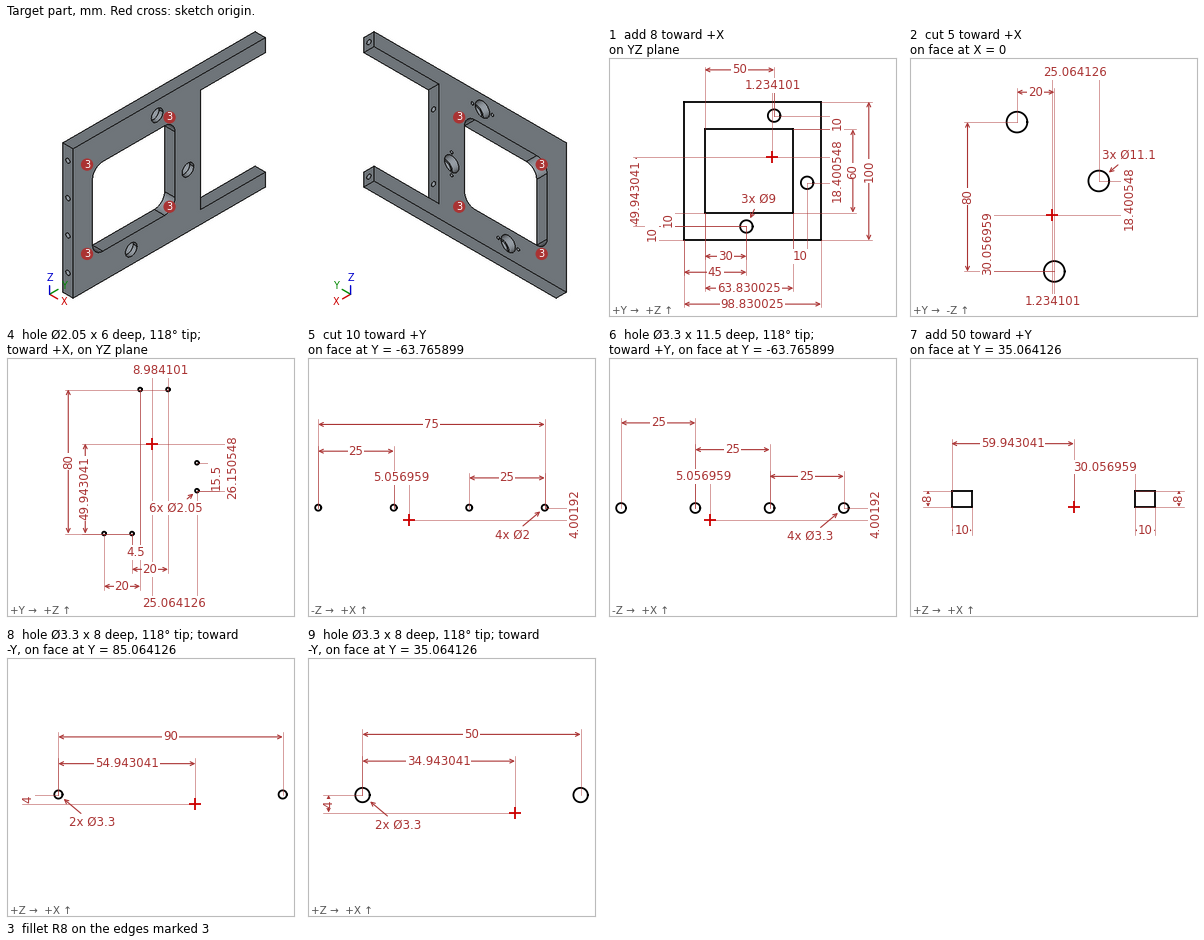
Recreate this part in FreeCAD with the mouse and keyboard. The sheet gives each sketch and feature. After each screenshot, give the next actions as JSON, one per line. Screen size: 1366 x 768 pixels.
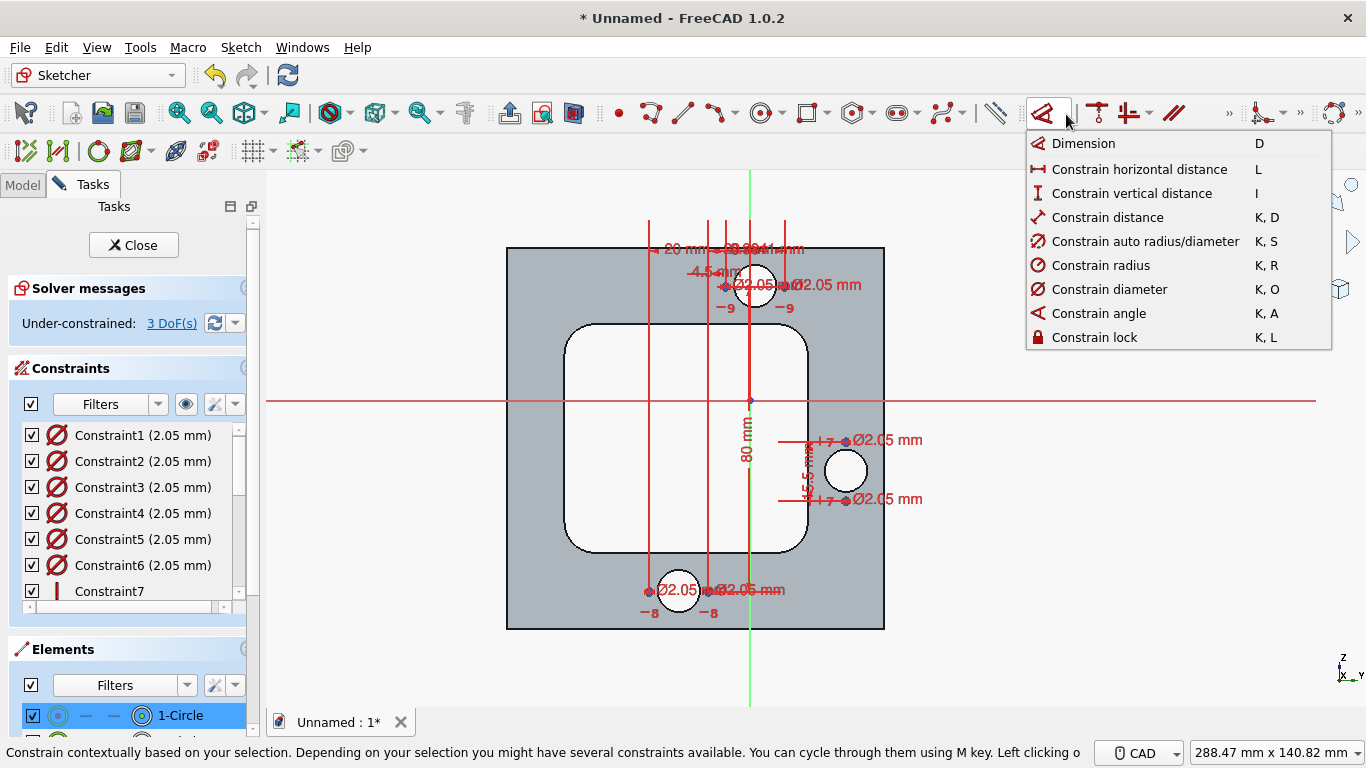
{"action": "left_click", "coordinate": [1179, 169]}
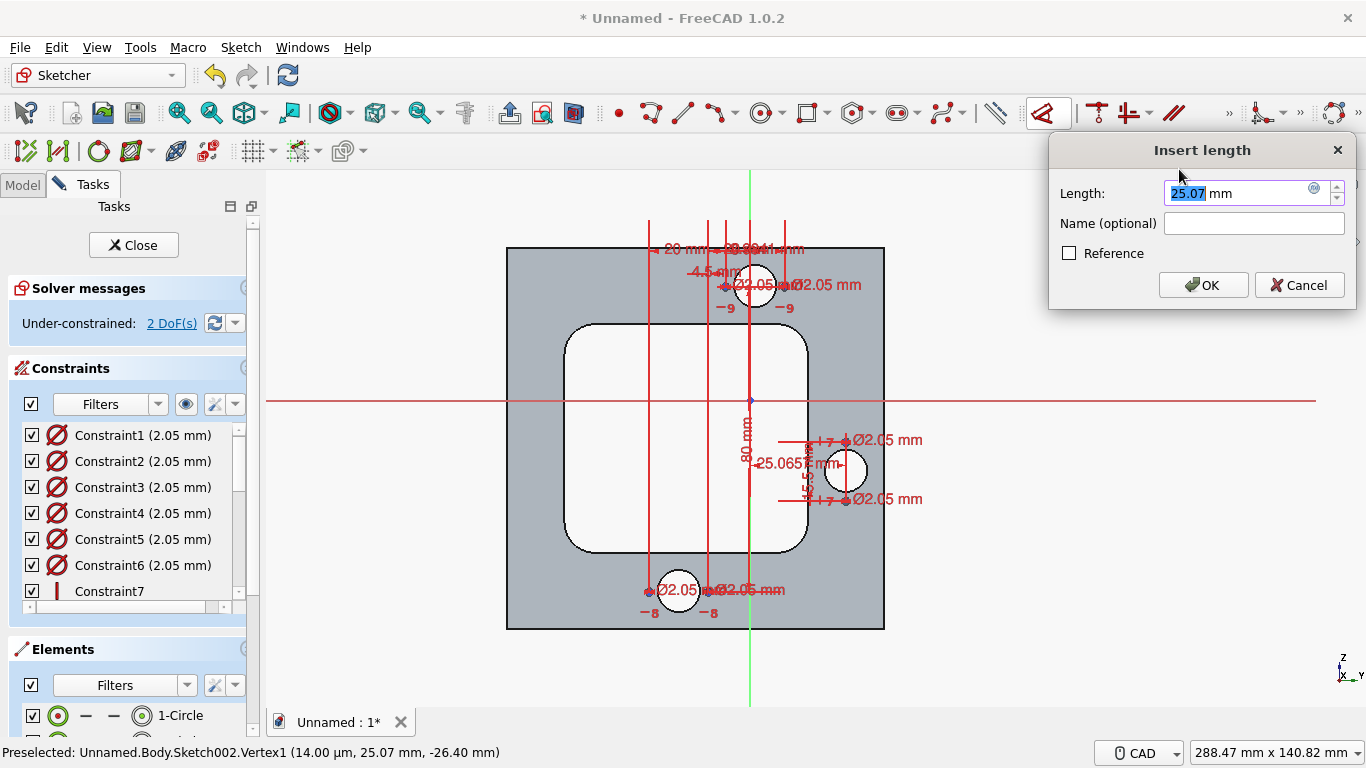
{"action": "type", "text": "25.064126"}
{"action": "key", "text": "Return"}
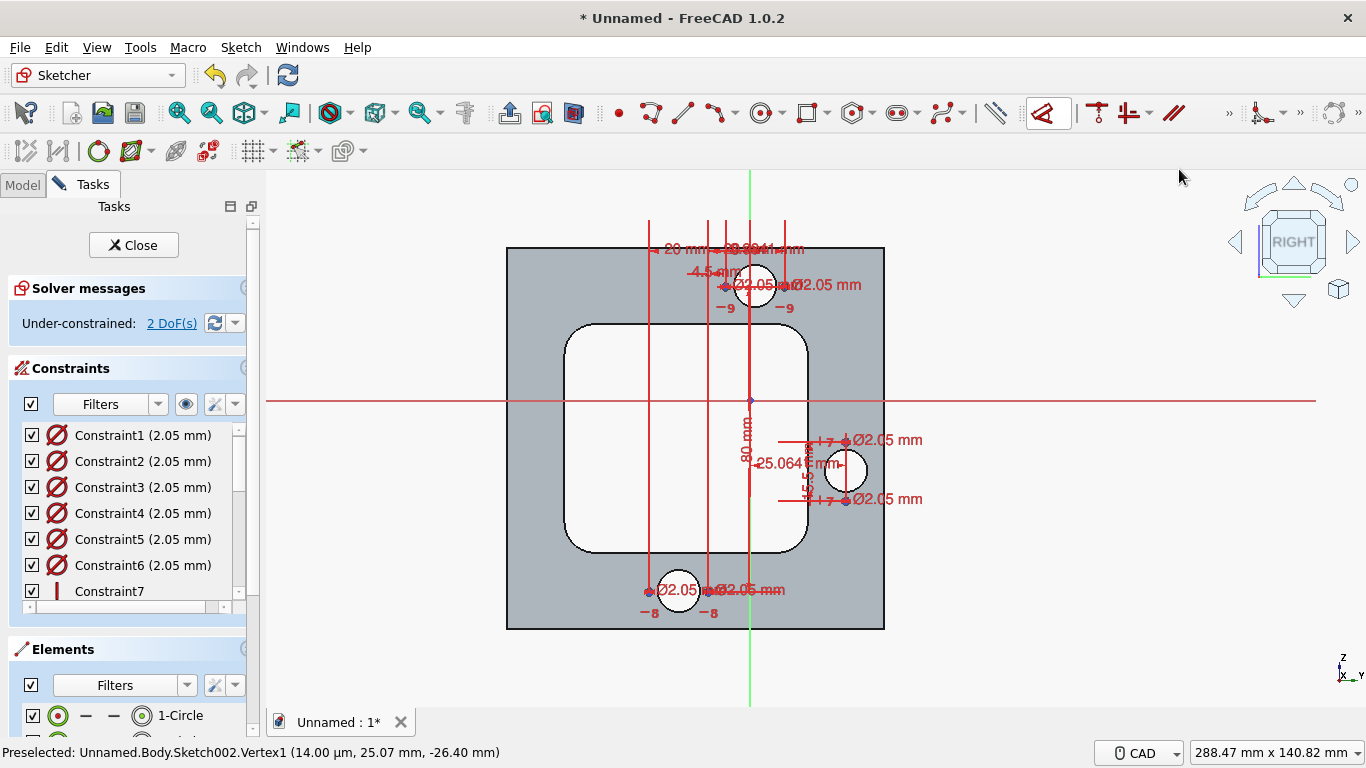
{"action": "left_click", "coordinate": [846, 501]}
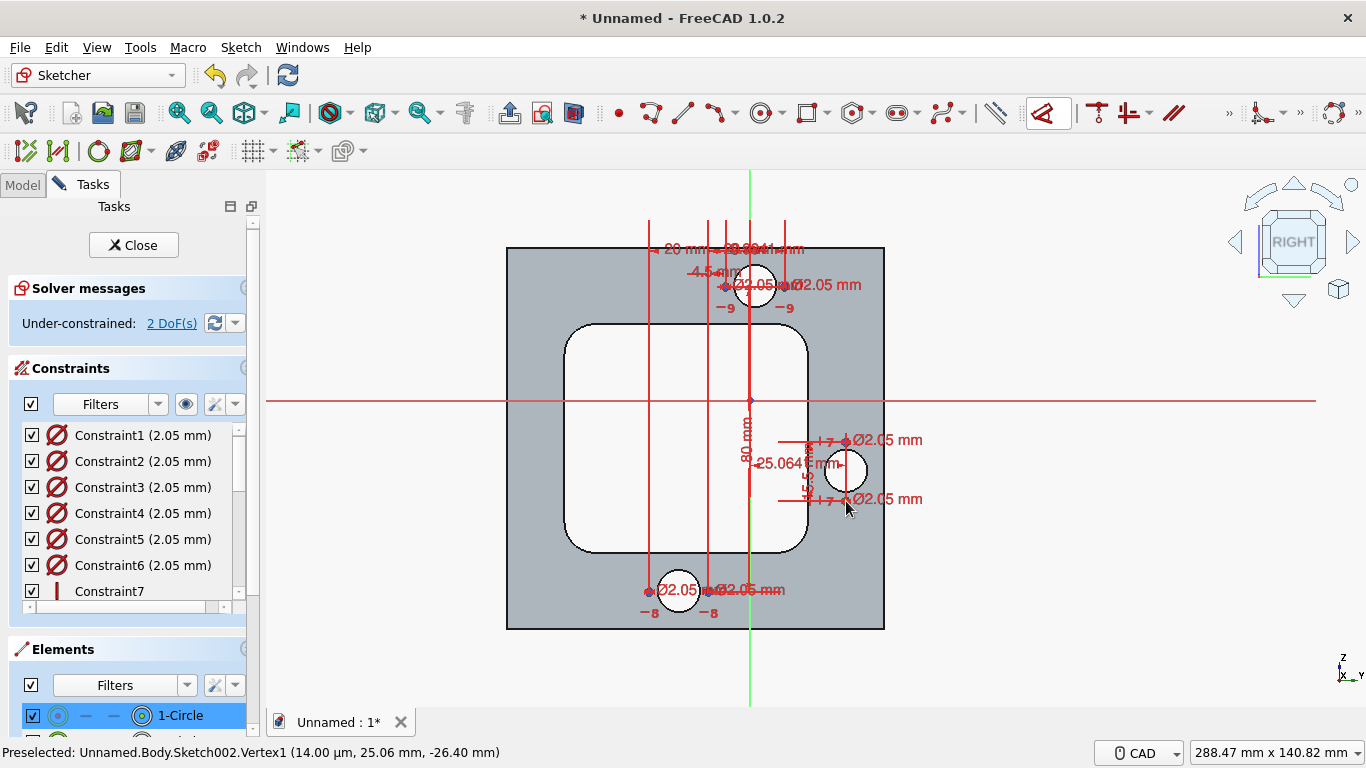
{"action": "key", "text": "i"}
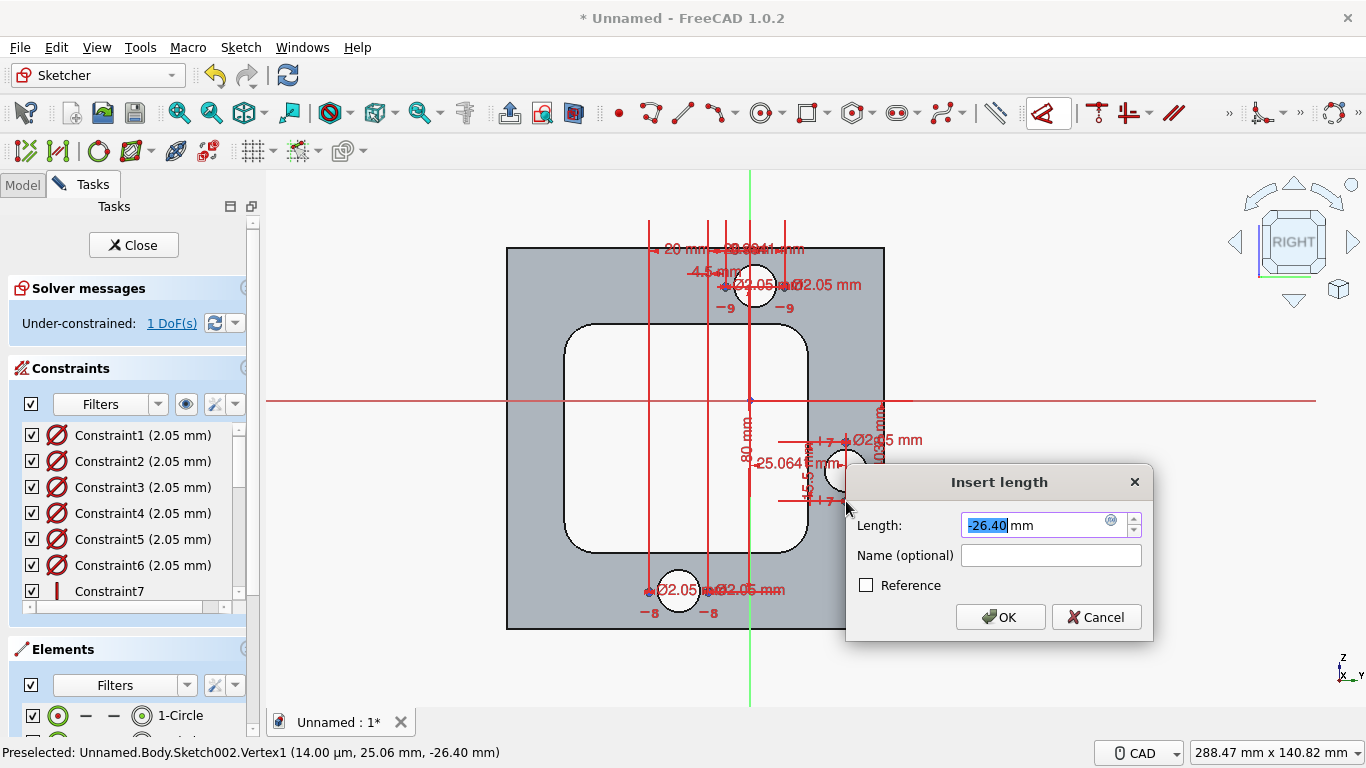
{"action": "type", "text": "-26.150548"}
{"action": "key", "text": "Return"}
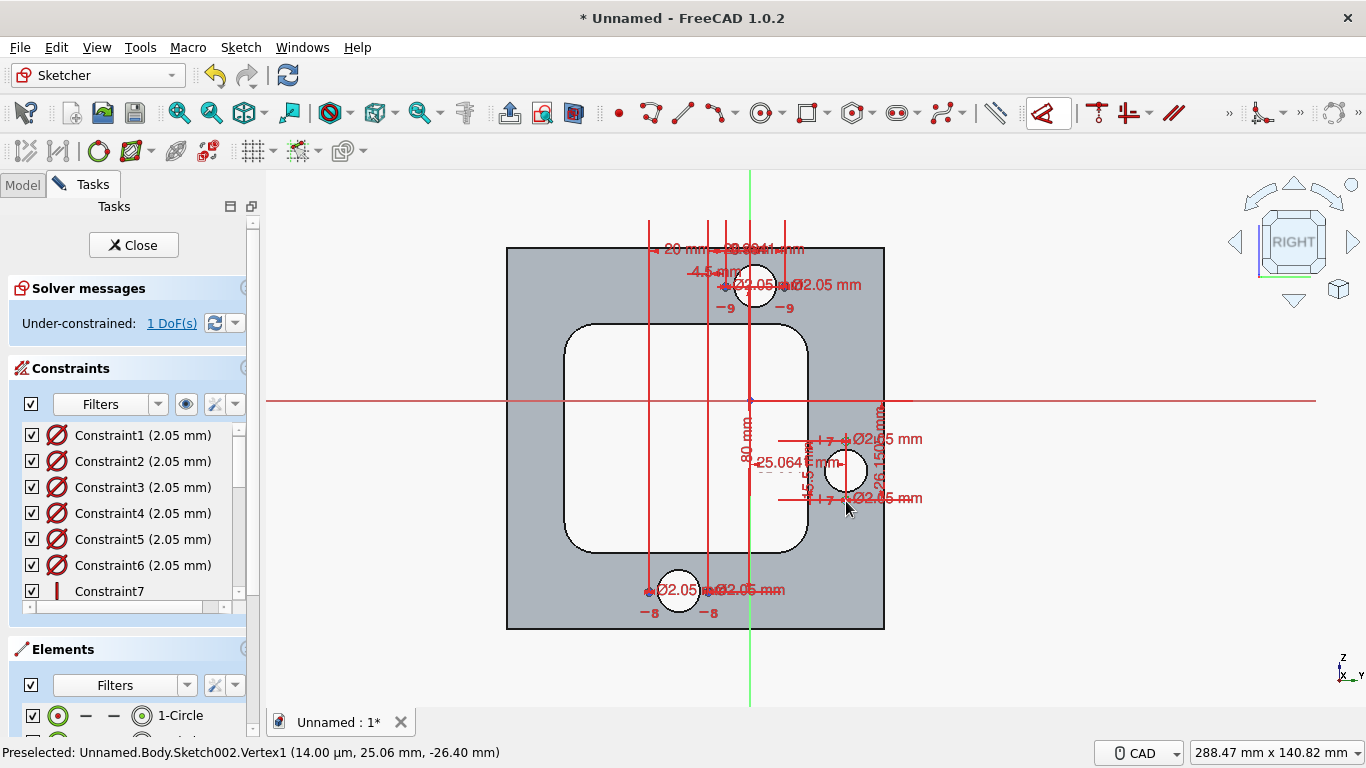
{"action": "left_click", "coordinate": [708, 592]}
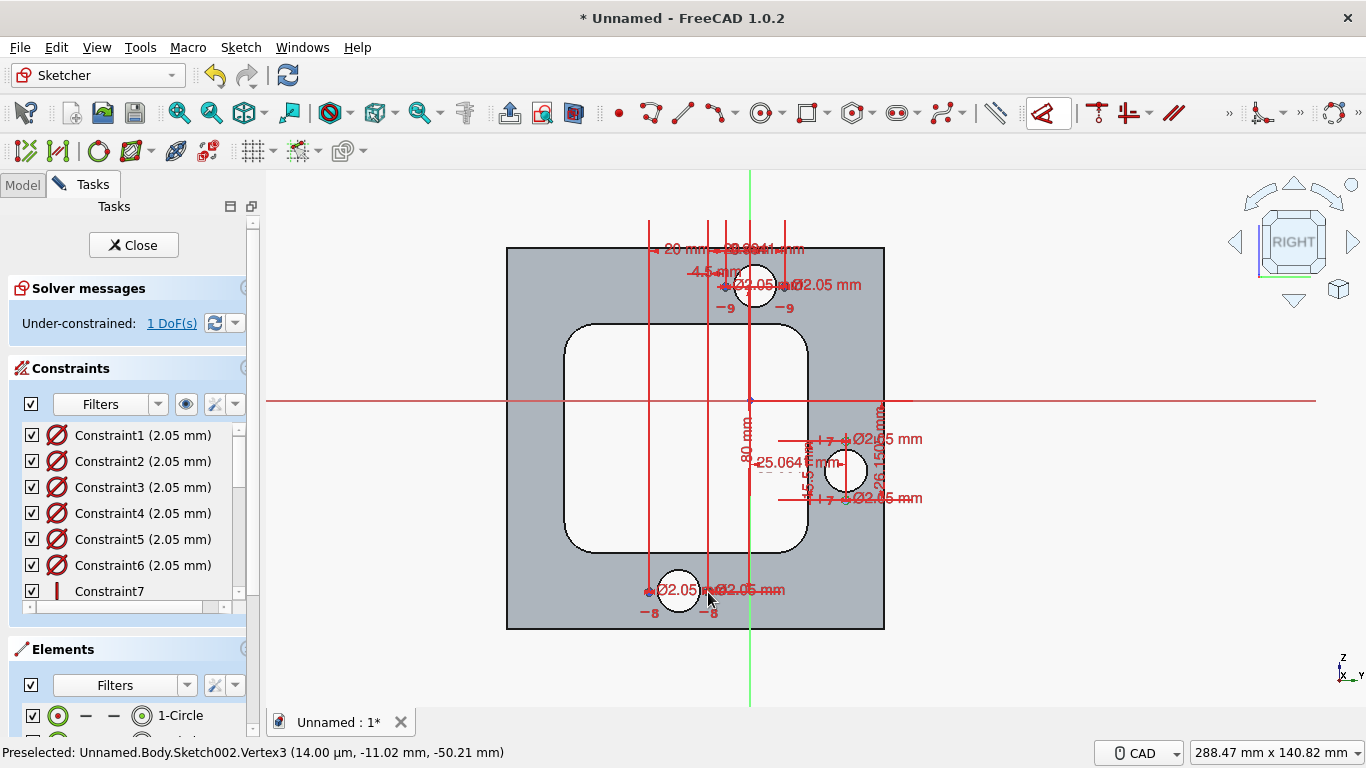
{"action": "key", "text": "i"}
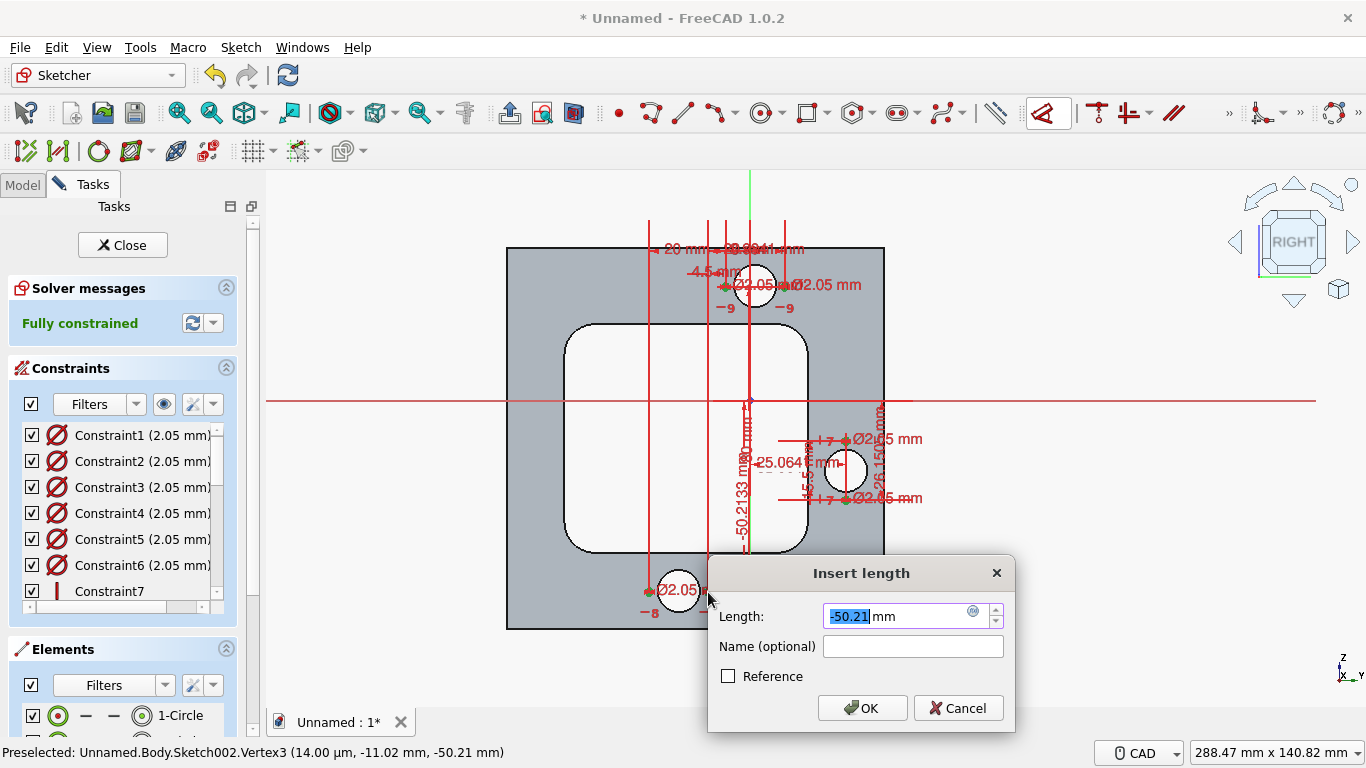
{"action": "type", "text": "-49.943041"}
{"action": "key", "text": "Return"}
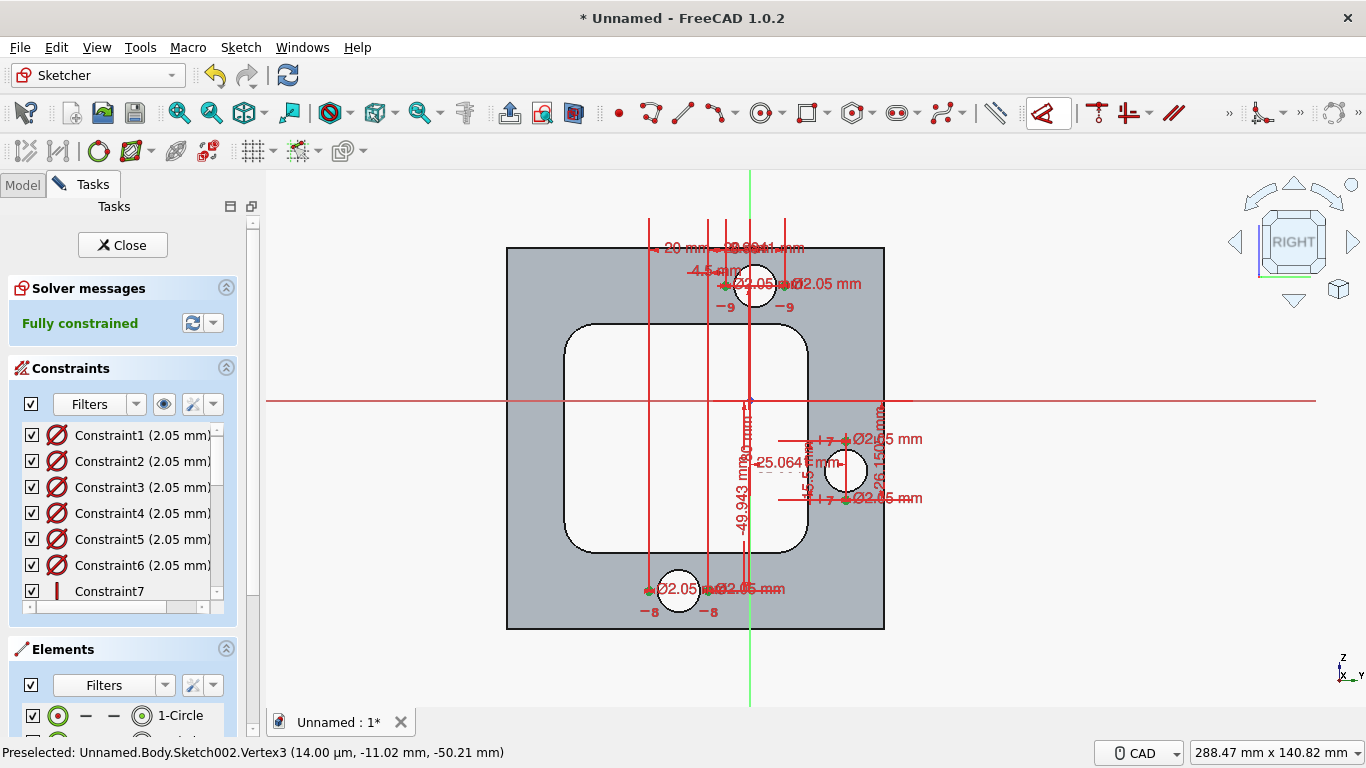
{"action": "left_click", "coordinate": [123, 245]}